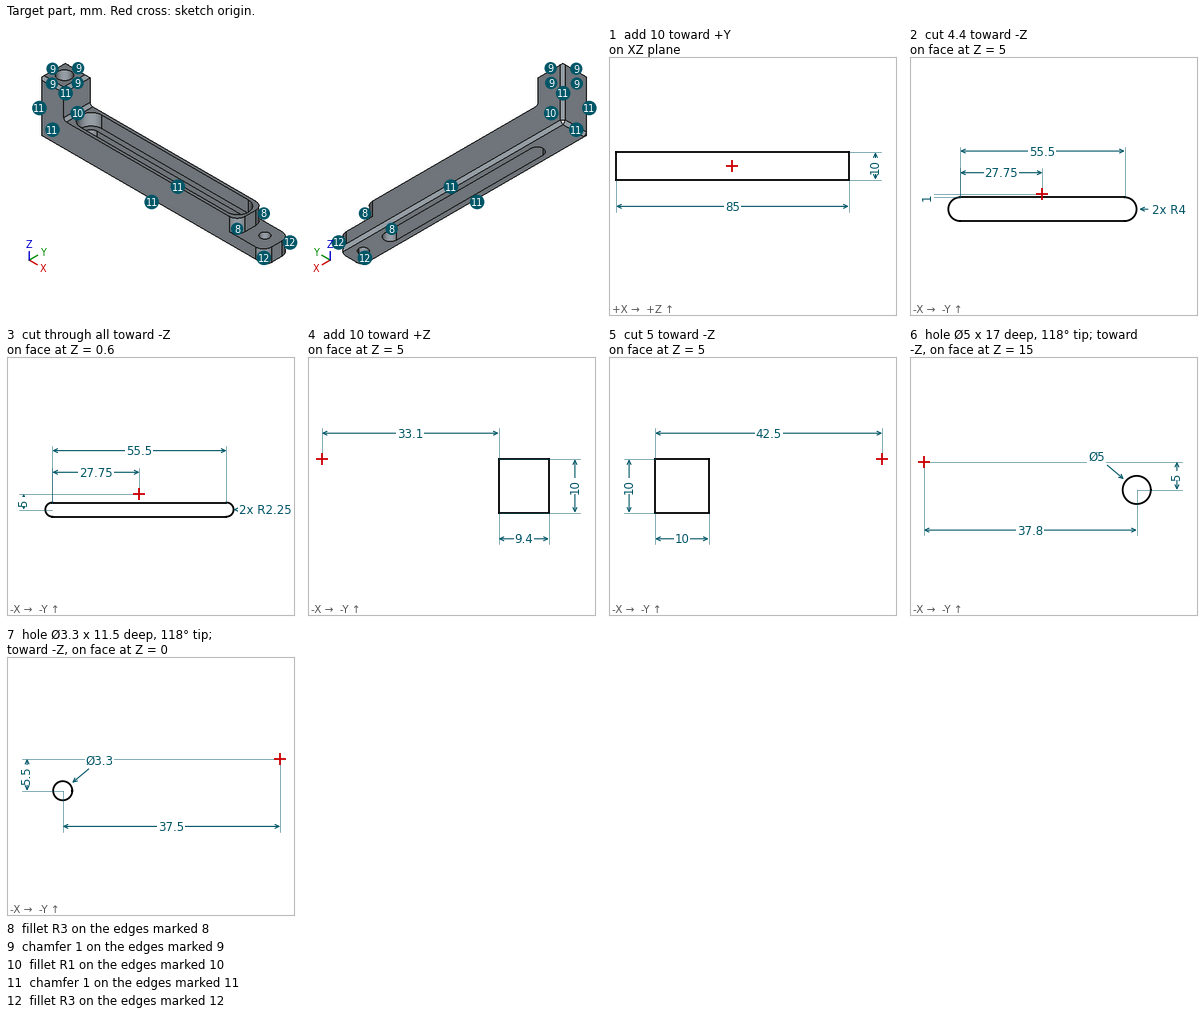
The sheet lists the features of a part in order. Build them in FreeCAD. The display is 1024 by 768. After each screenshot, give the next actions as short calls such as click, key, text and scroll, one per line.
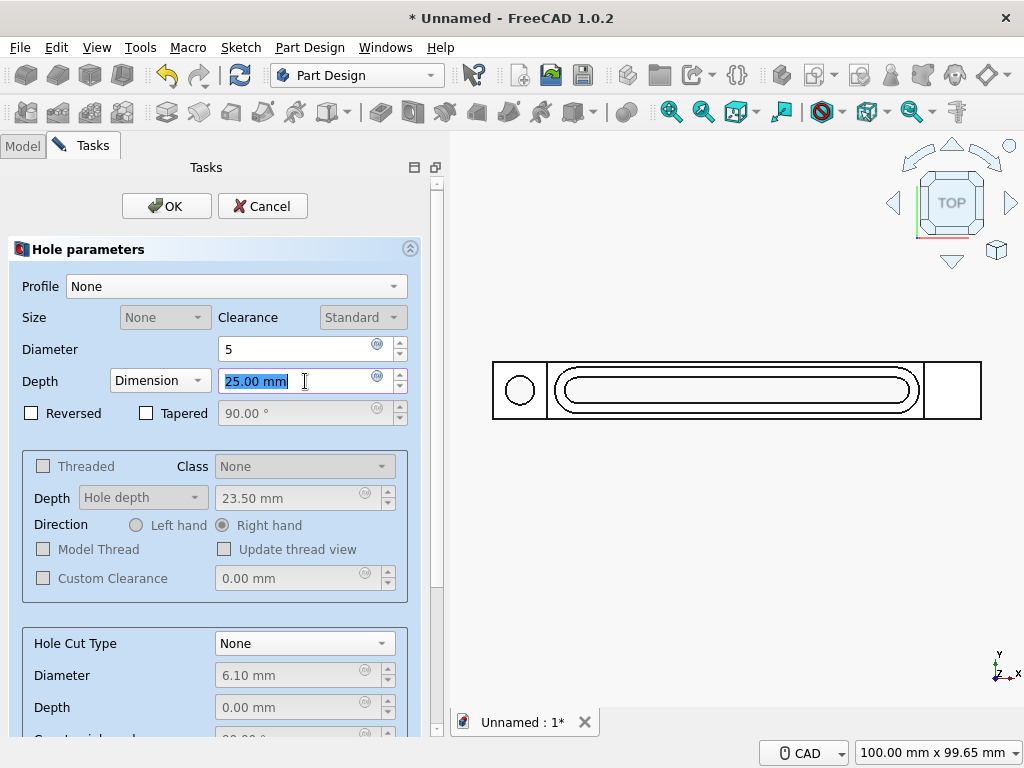
text(17)
key(Tab)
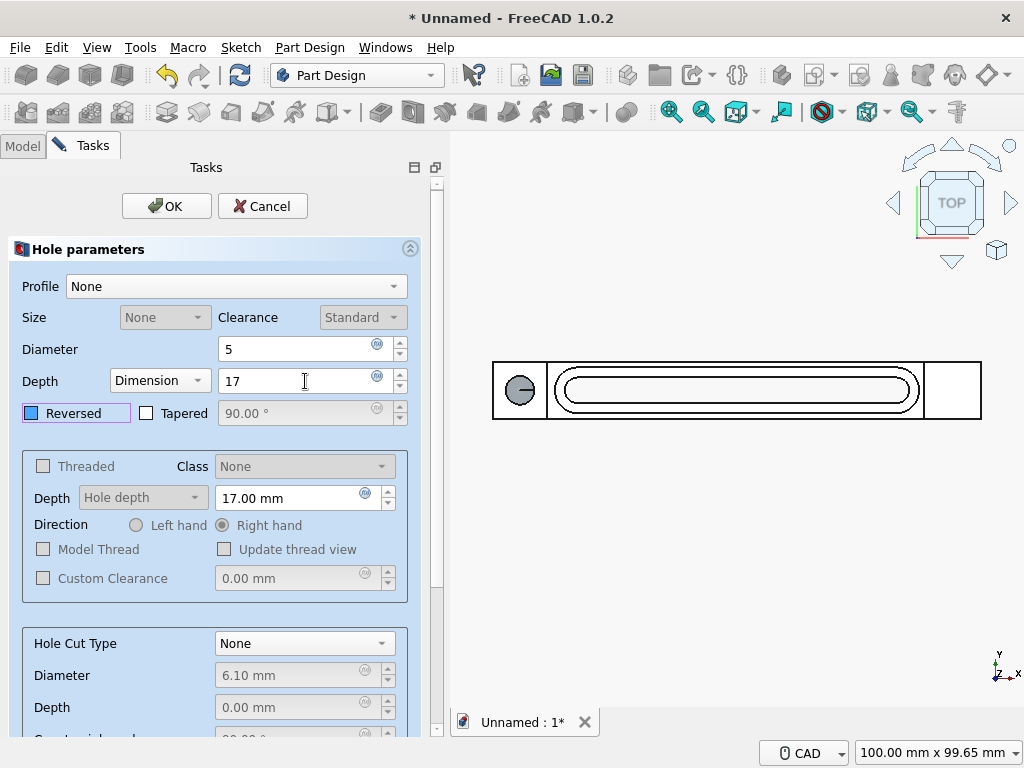
click(167, 206)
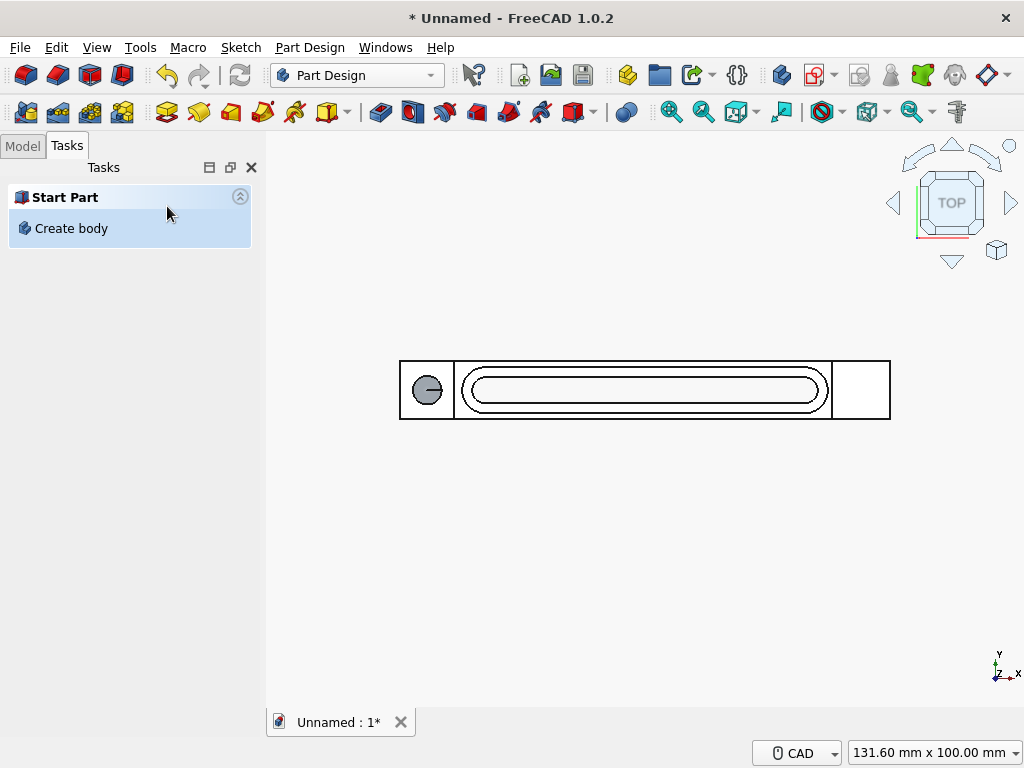
click(861, 389)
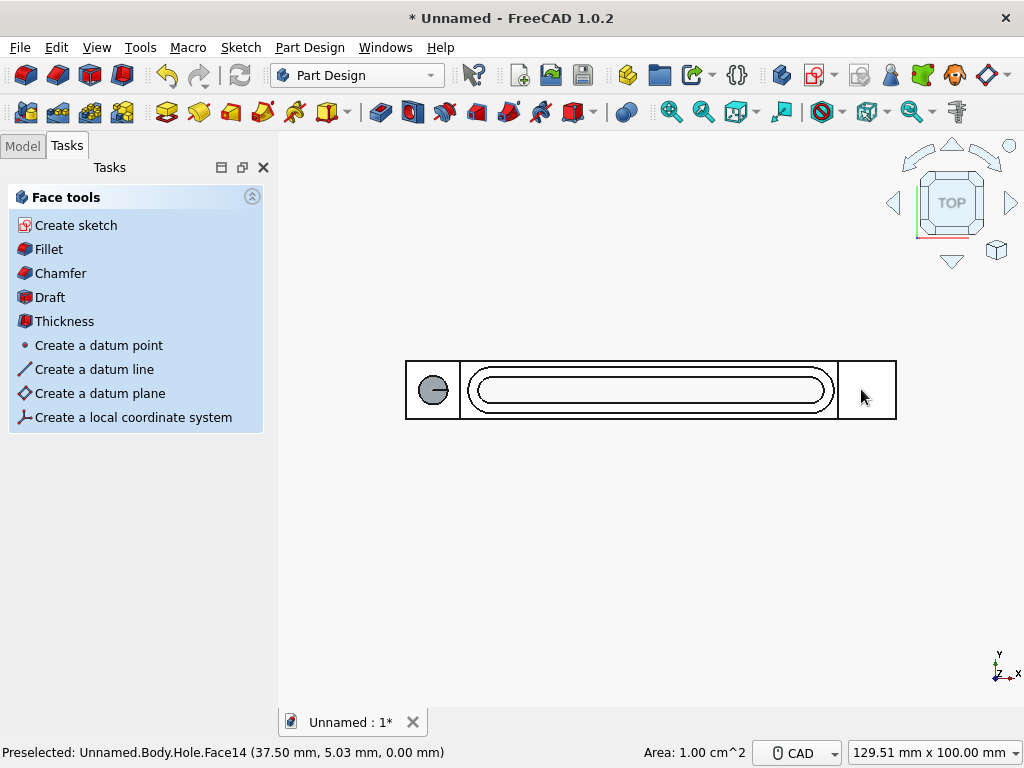
click(814, 76)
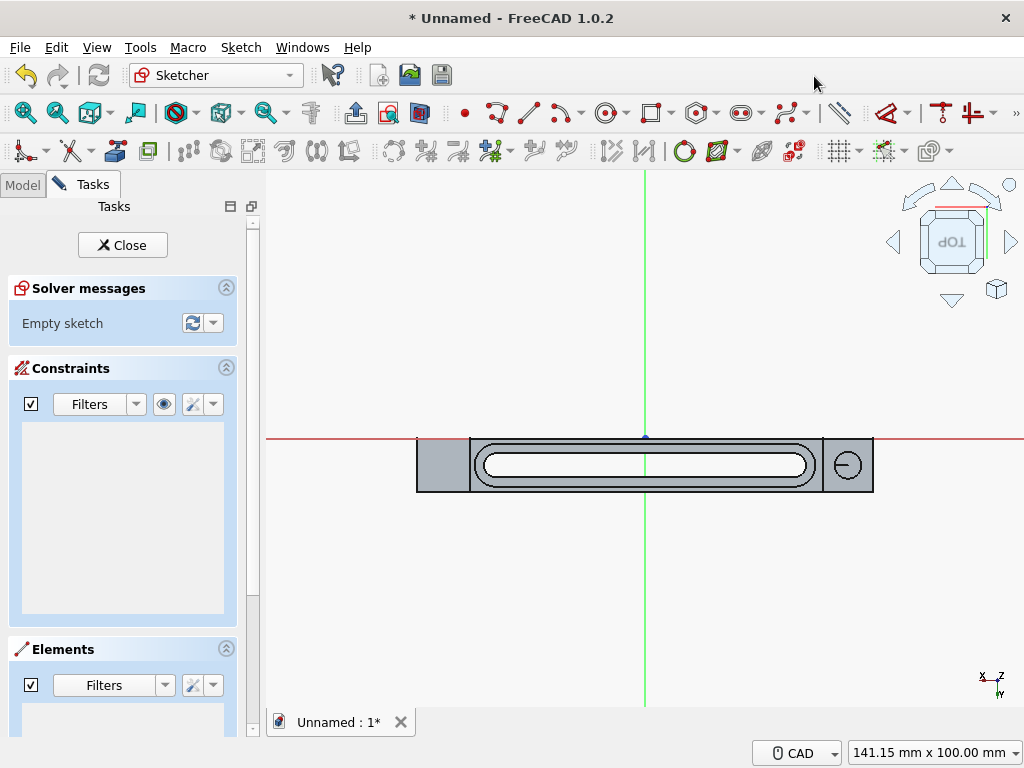
scroll(437, 470, up, 15)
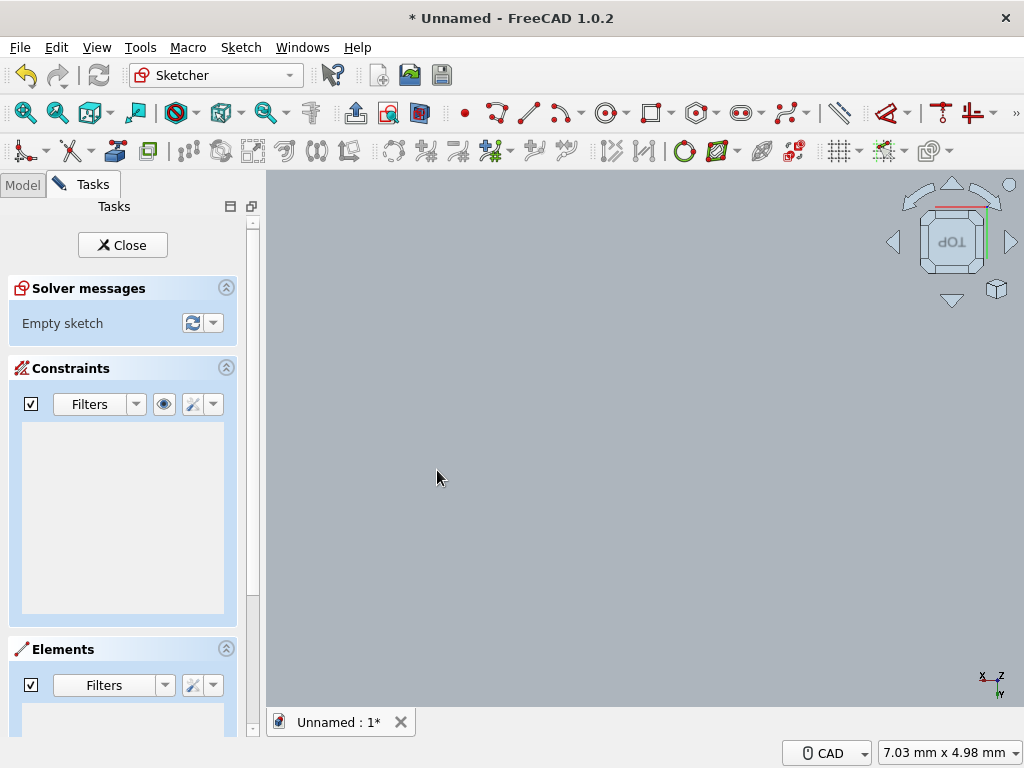
key(g)
key(c)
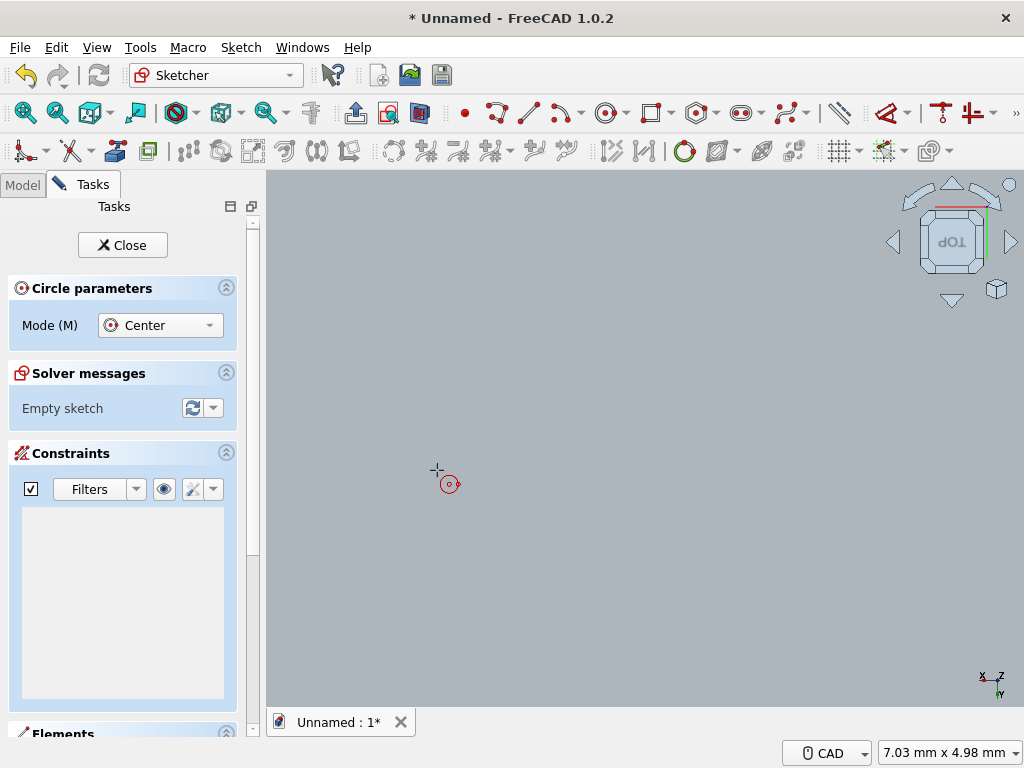
click(566, 420)
click(692, 294)
key(Escape)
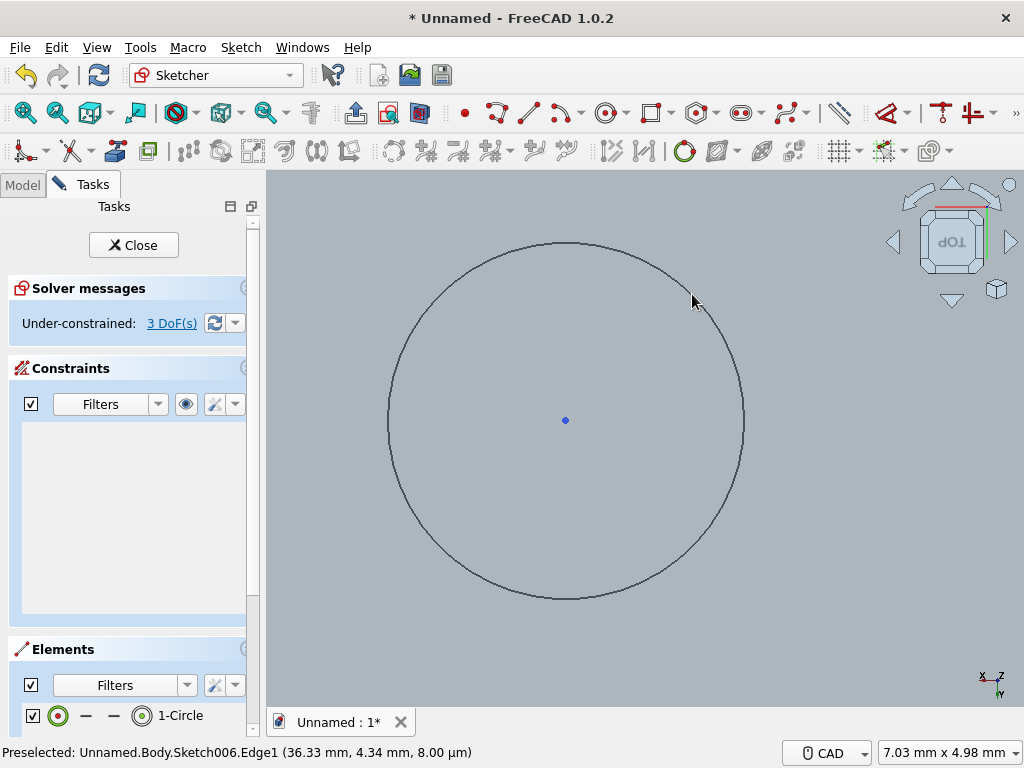
key(d)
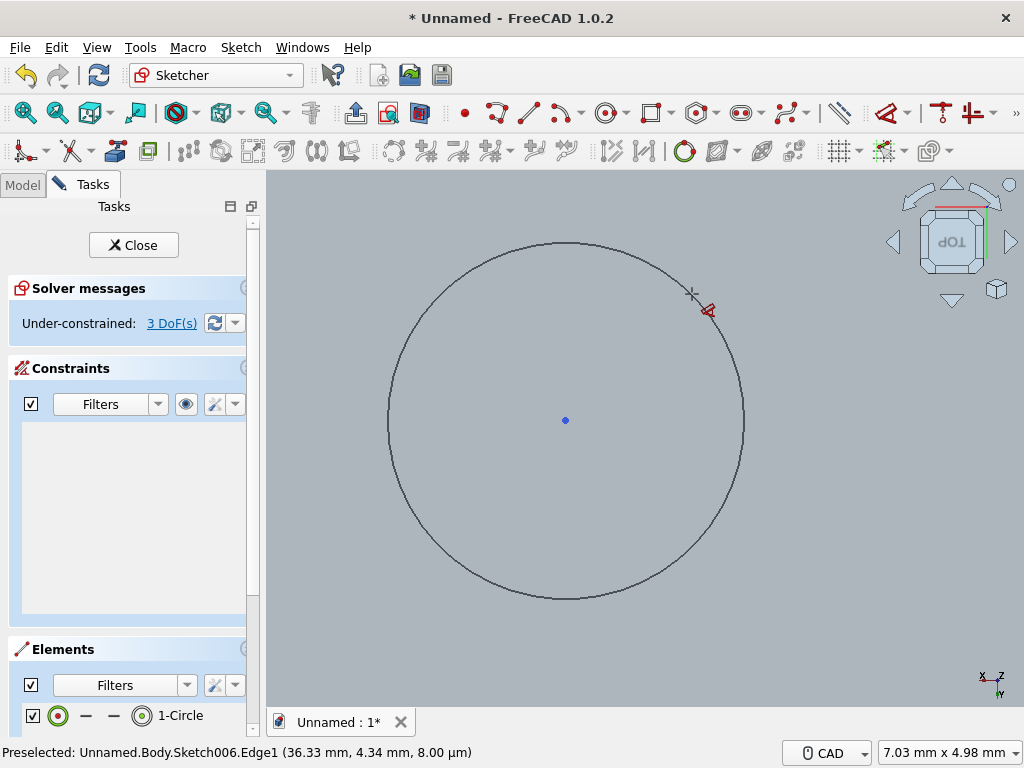
click(692, 295)
click(715, 272)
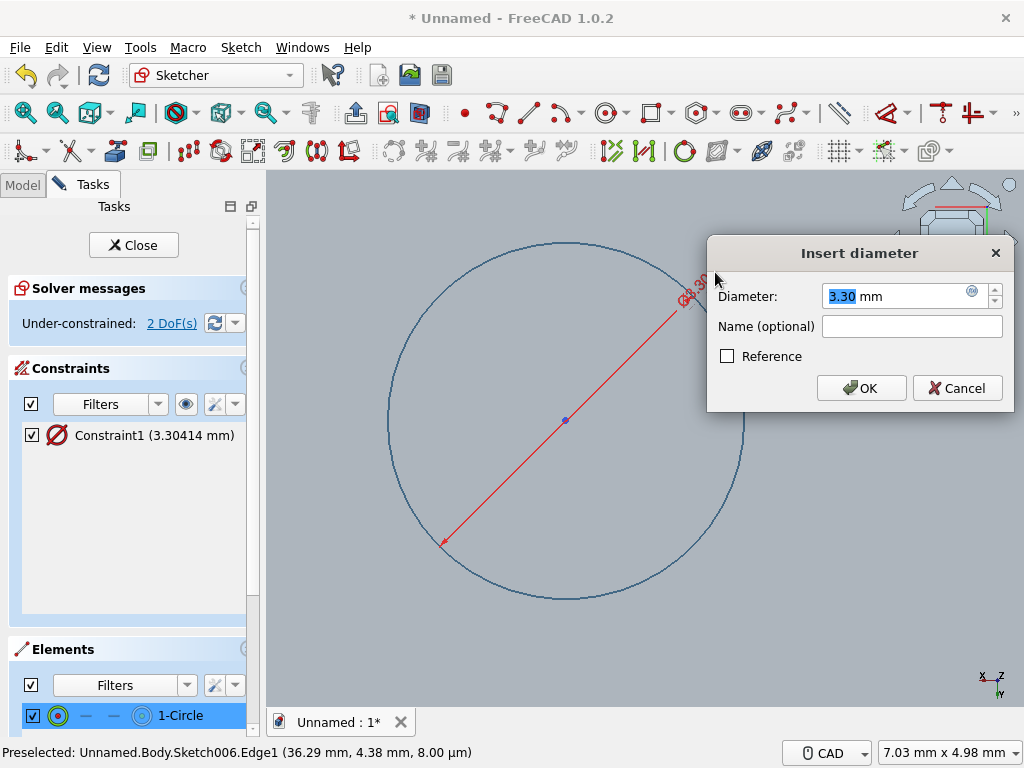
text(3.3)
key(Return)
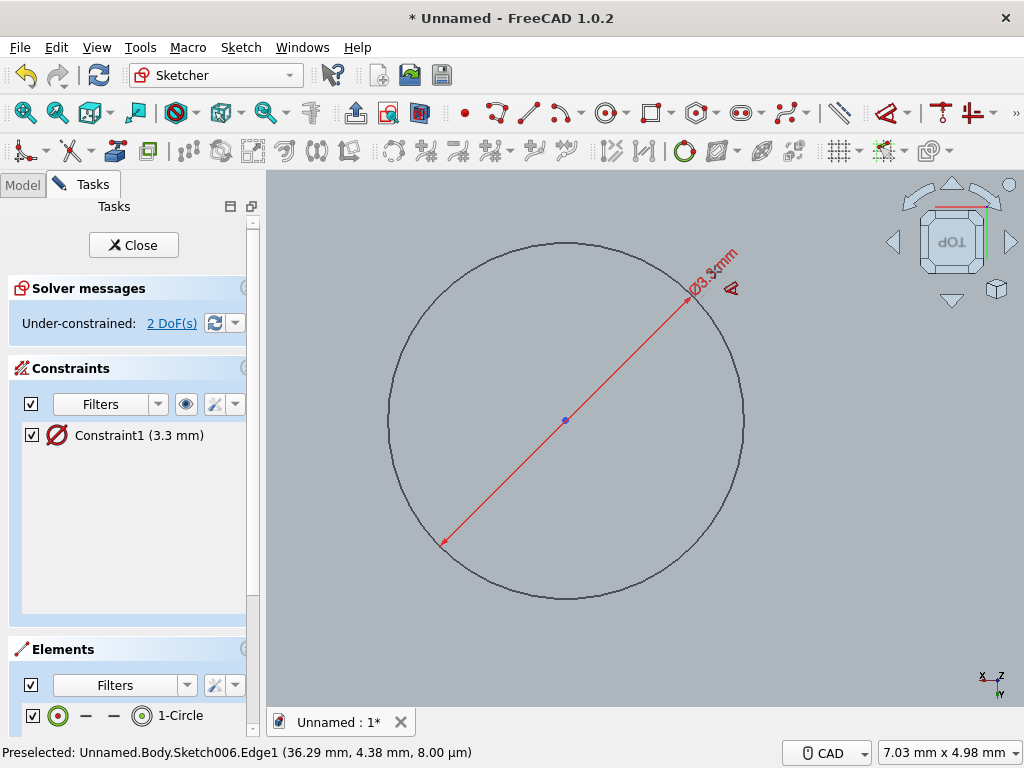
click(566, 421)
click(532, 309)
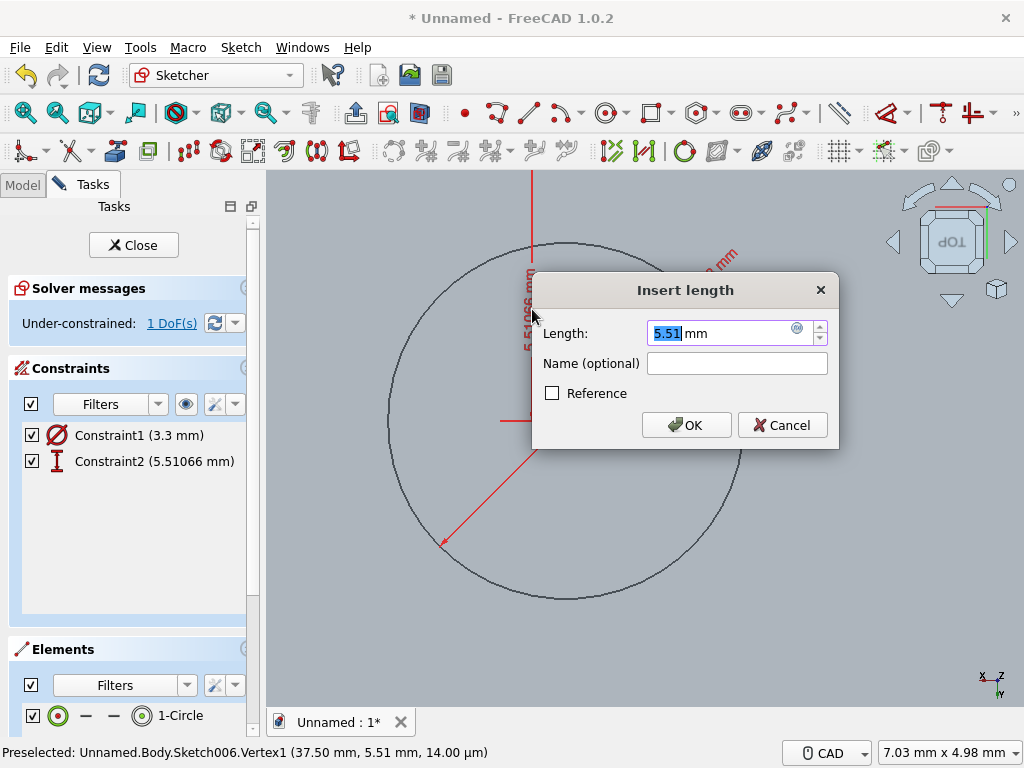
text(5.5)
key(Return)